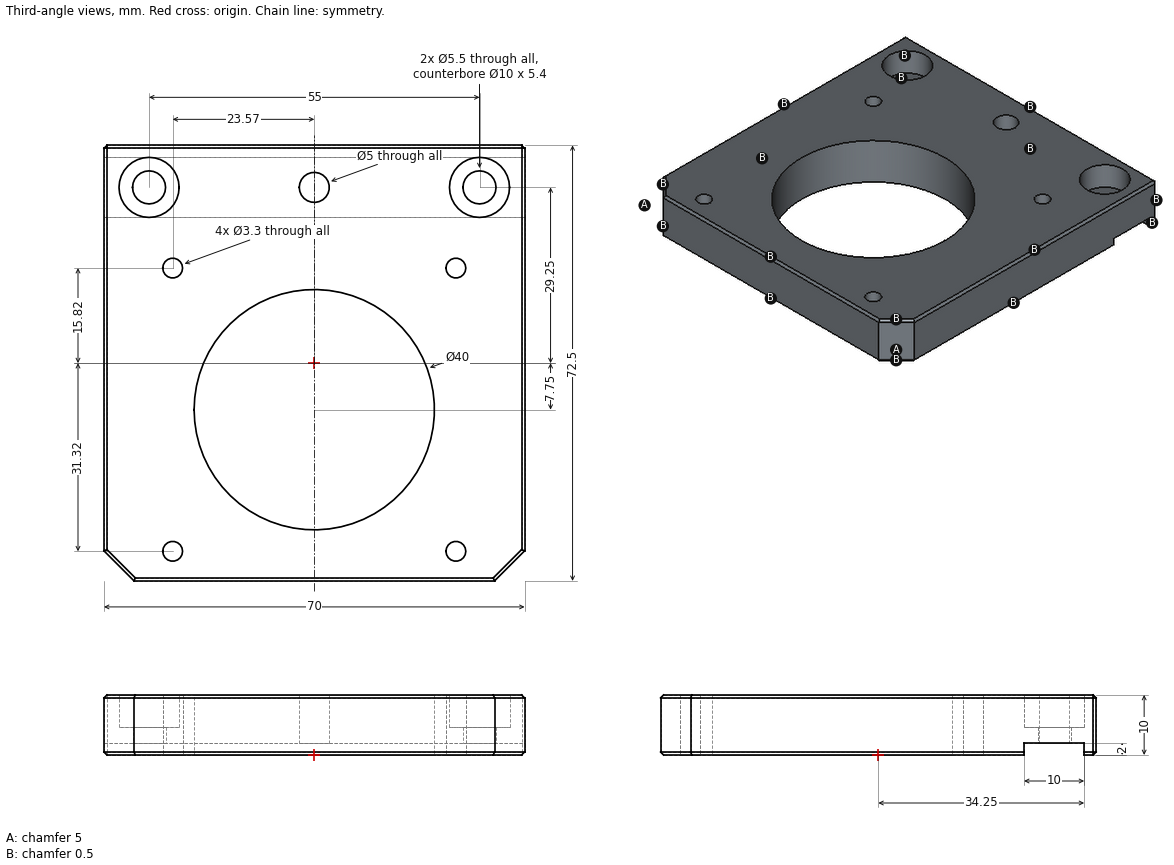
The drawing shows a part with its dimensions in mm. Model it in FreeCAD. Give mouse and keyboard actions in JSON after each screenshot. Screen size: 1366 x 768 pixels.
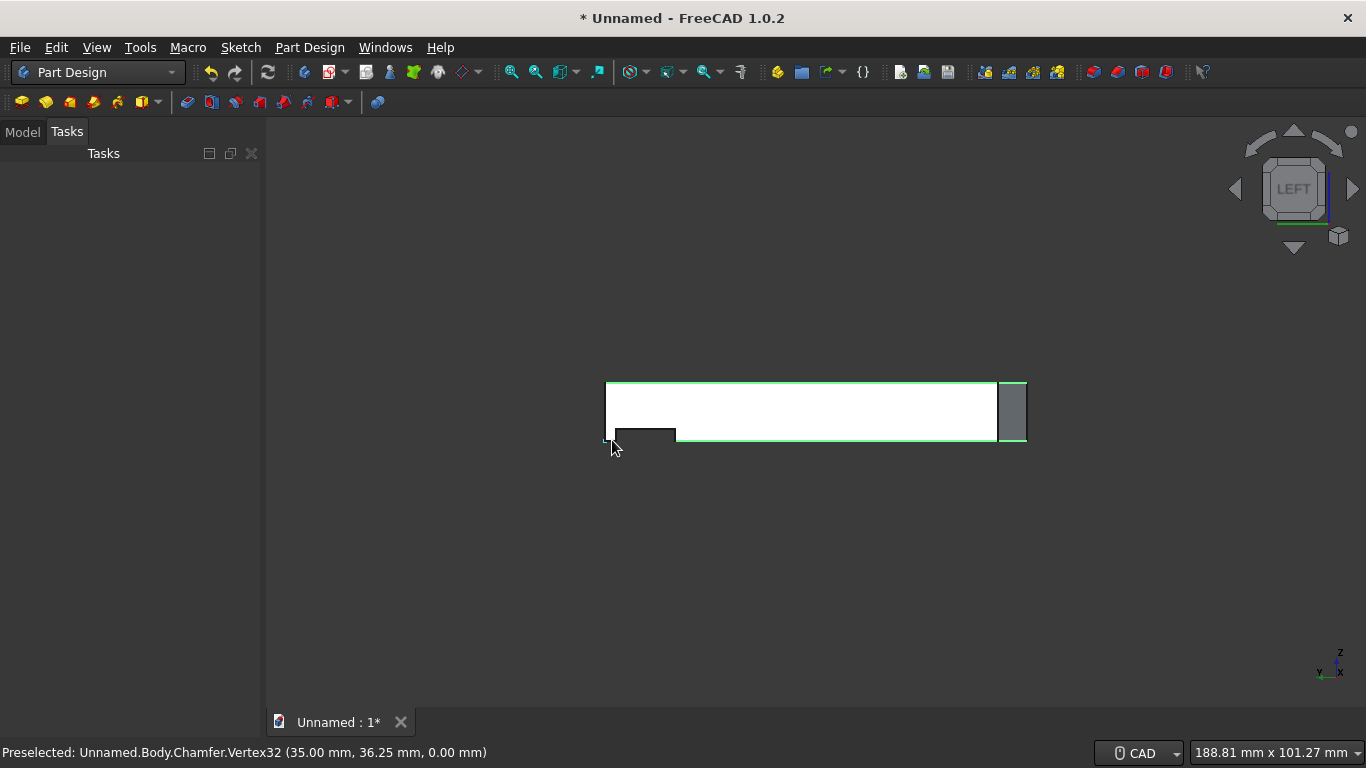
{"action": "left_click", "coordinate": [512, 72]}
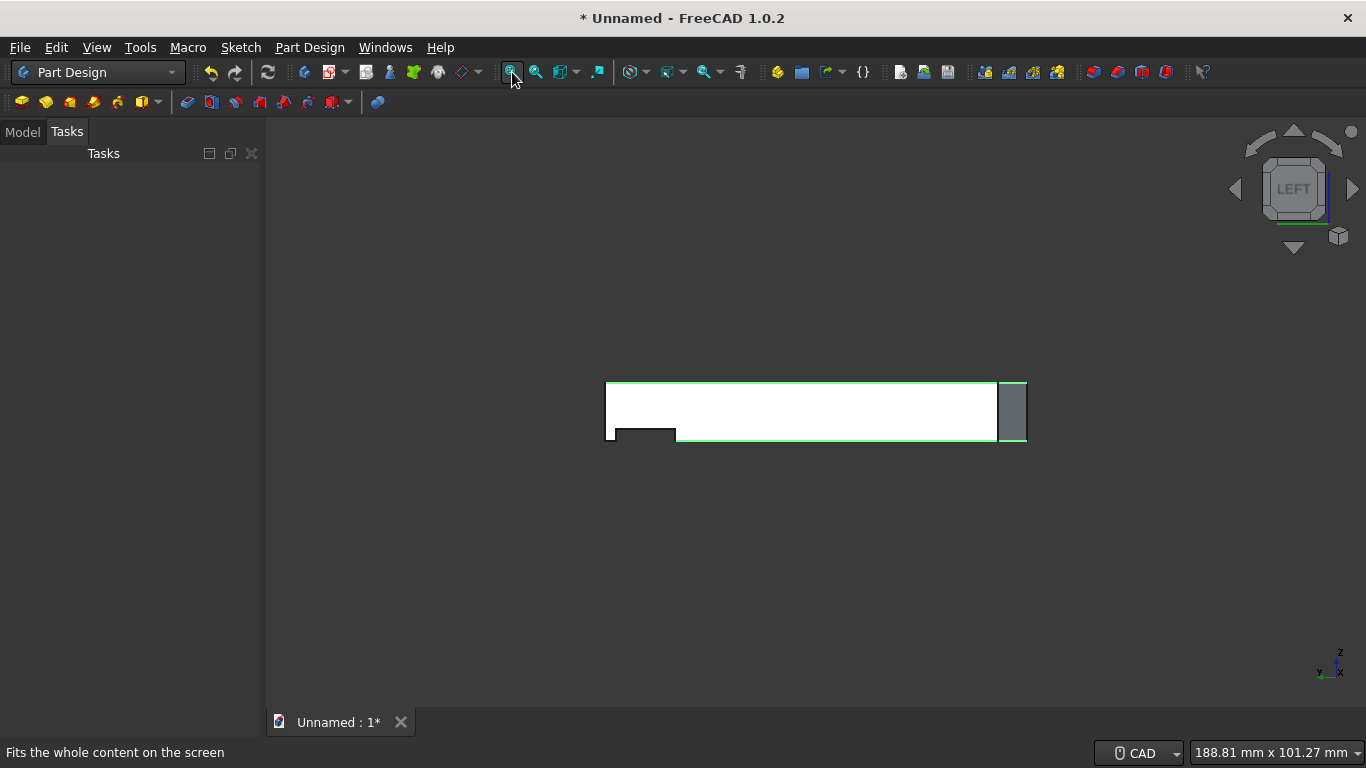
{"action": "scroll", "coordinate": [611, 440], "scroll_direction": "up", "scroll_amount": 7}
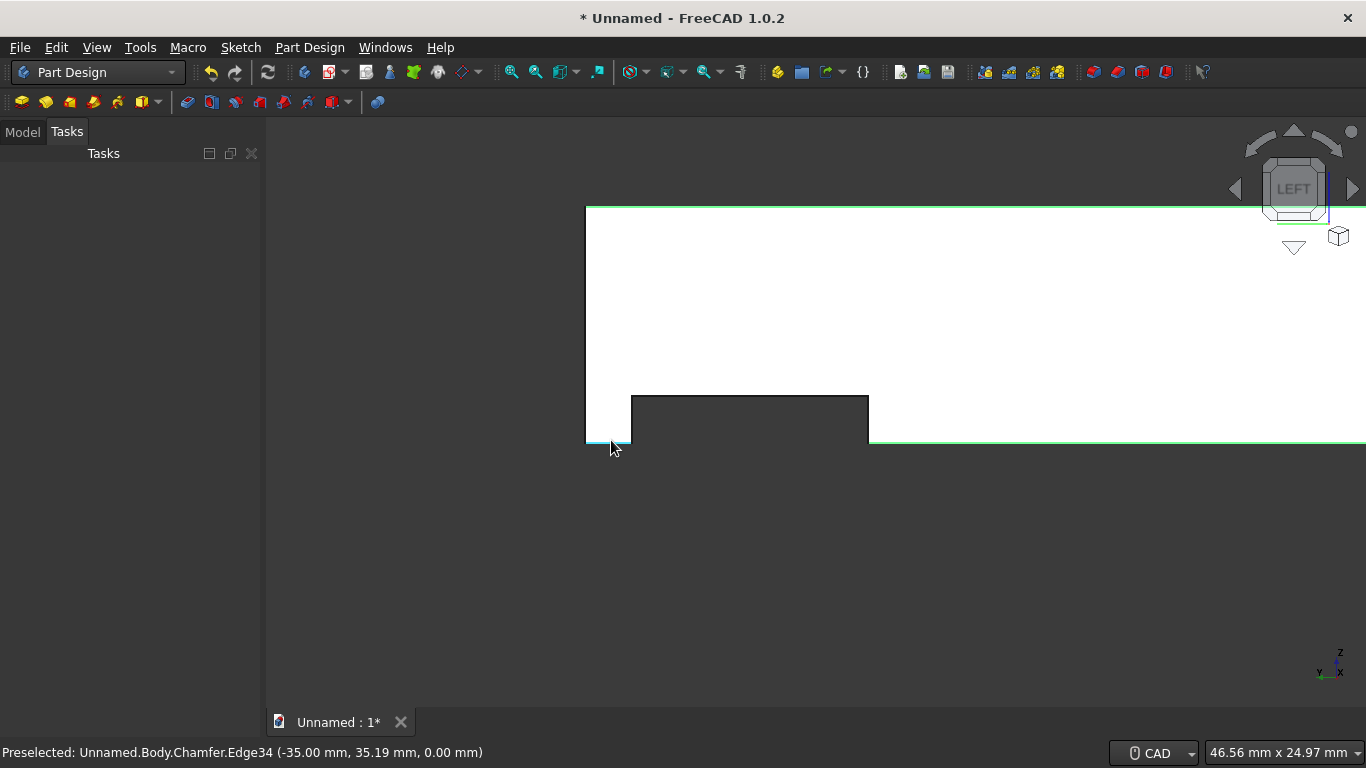
{"action": "left_click", "coordinate": [609, 442], "text": "ctrl"}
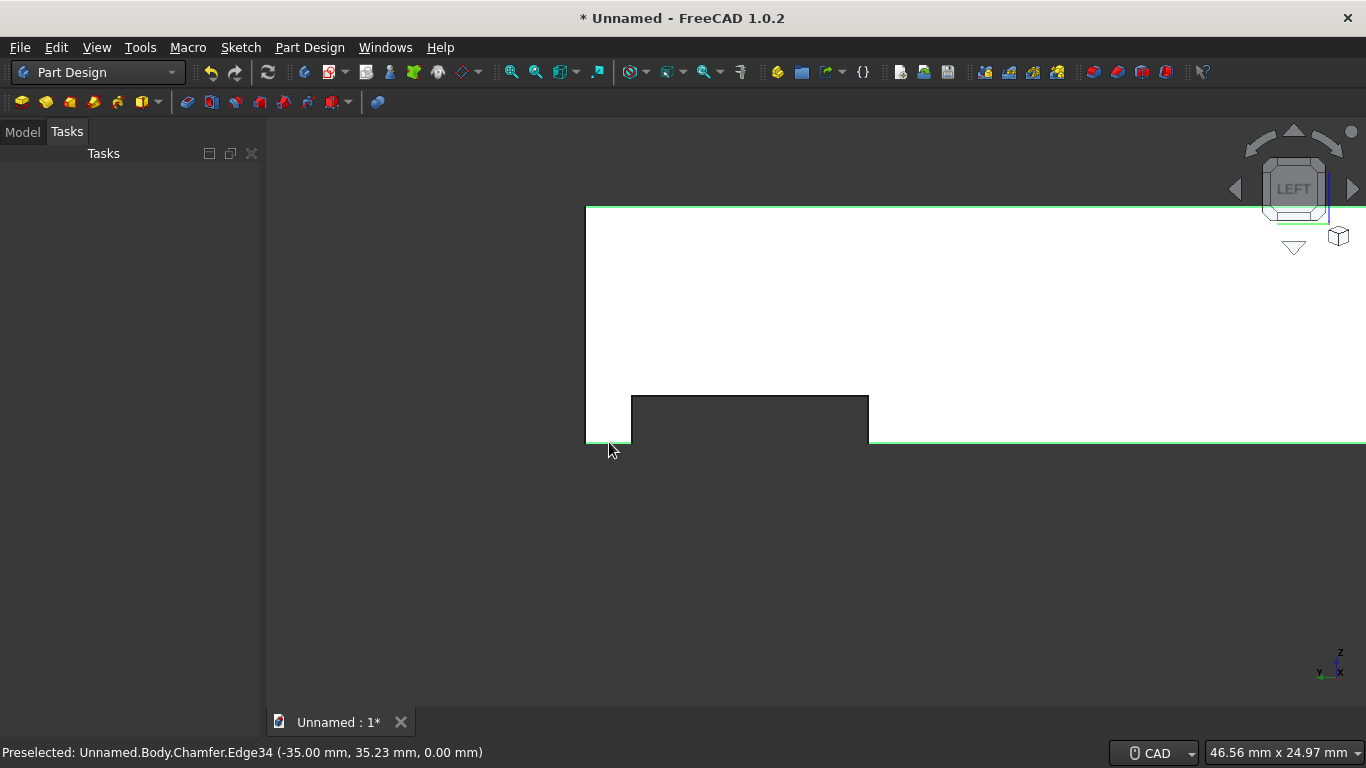
{"action": "left_click", "coordinate": [512, 72]}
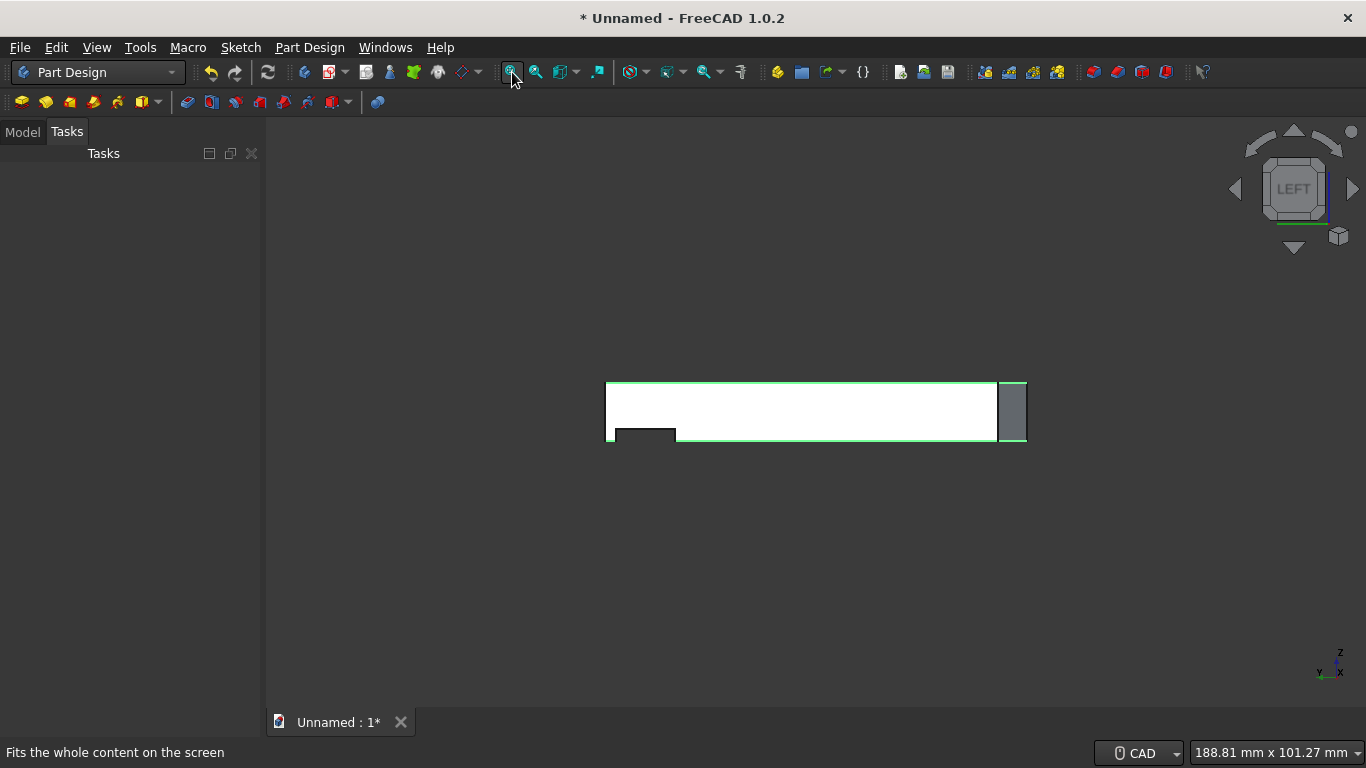
{"action": "key", "text": "v 3"}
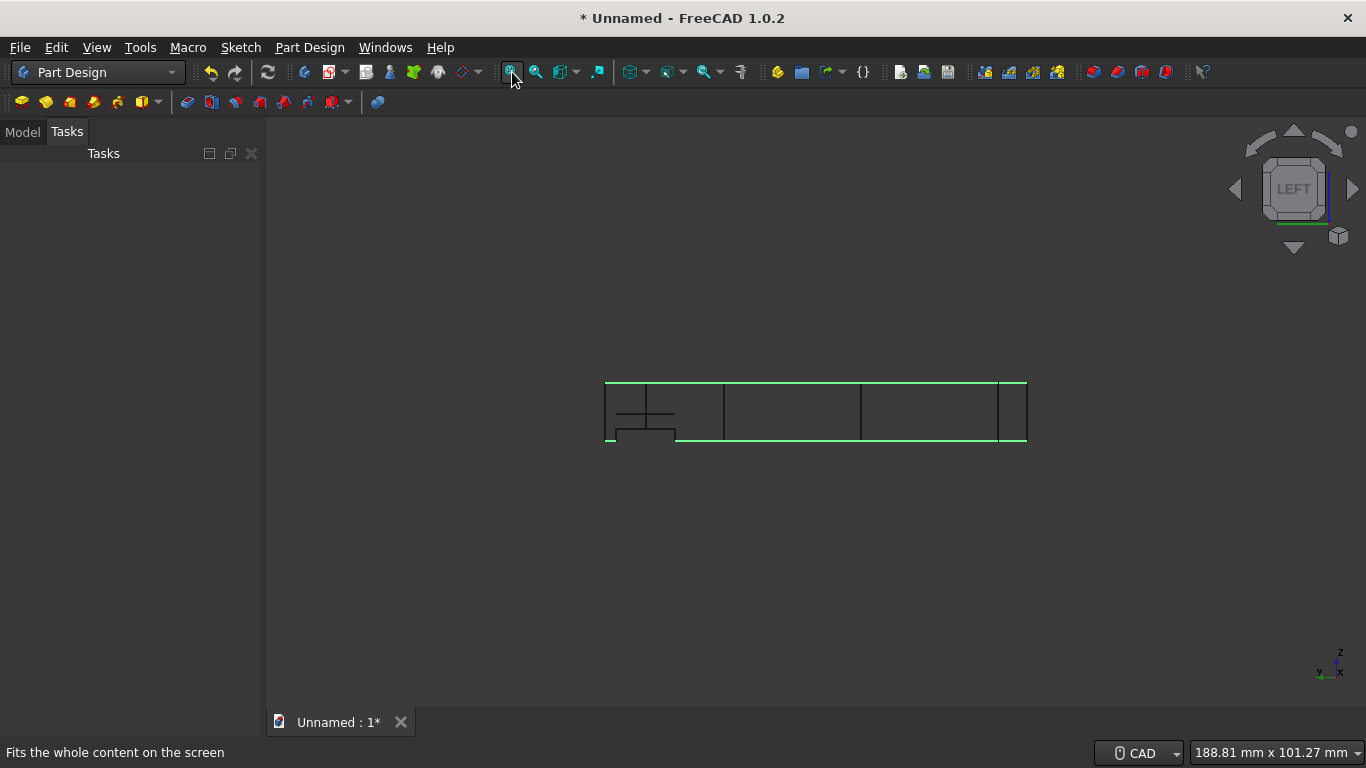
{"action": "key", "text": "0"}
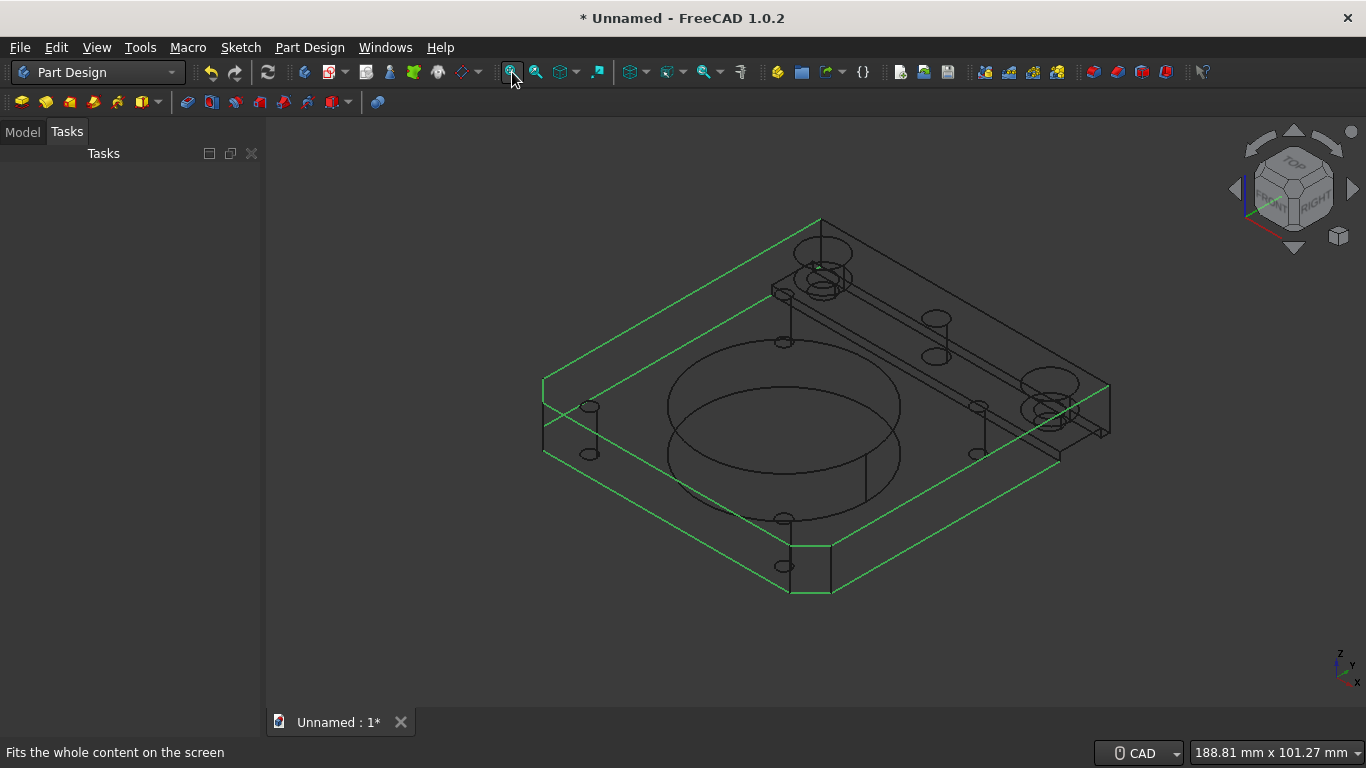
{"action": "scroll", "coordinate": [1105, 434], "scroll_direction": "up", "scroll_amount": 7}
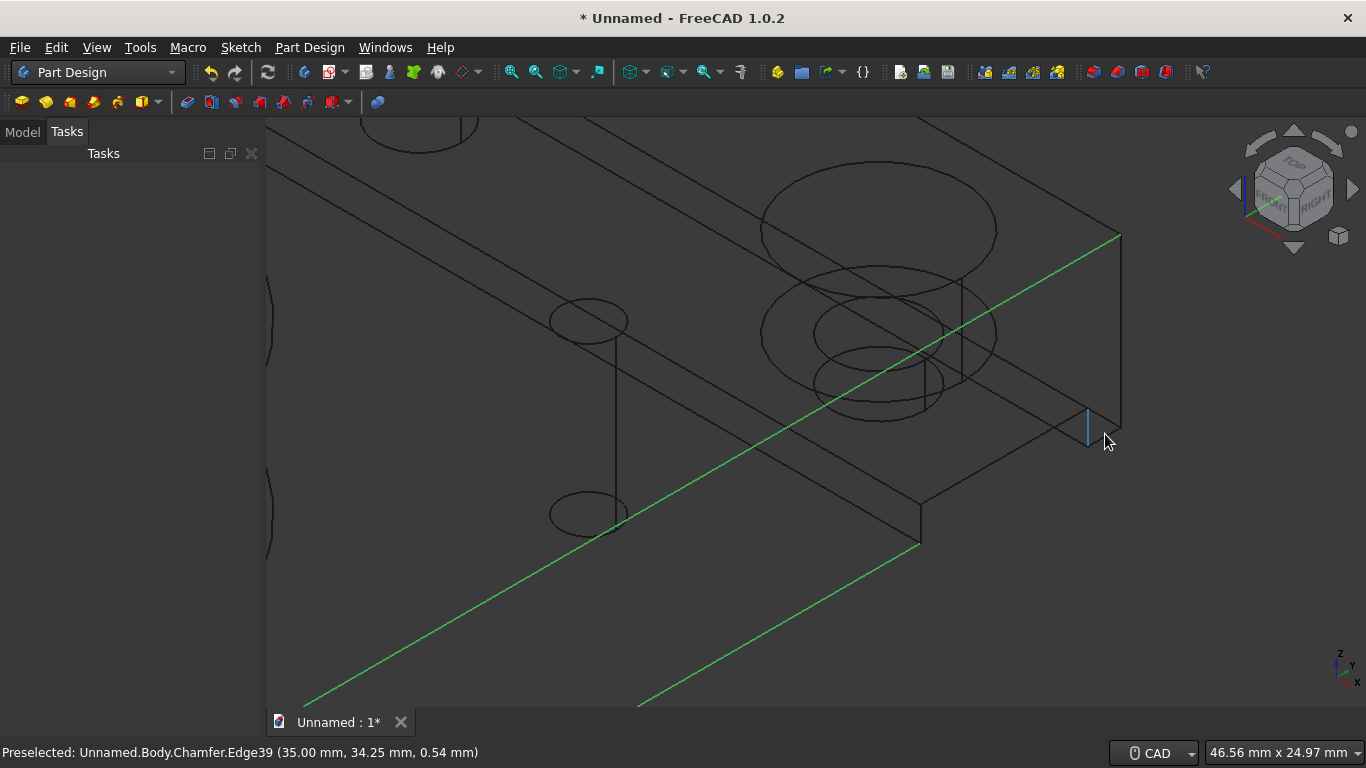
{"action": "left_click", "coordinate": [1104, 436], "text": "ctrl"}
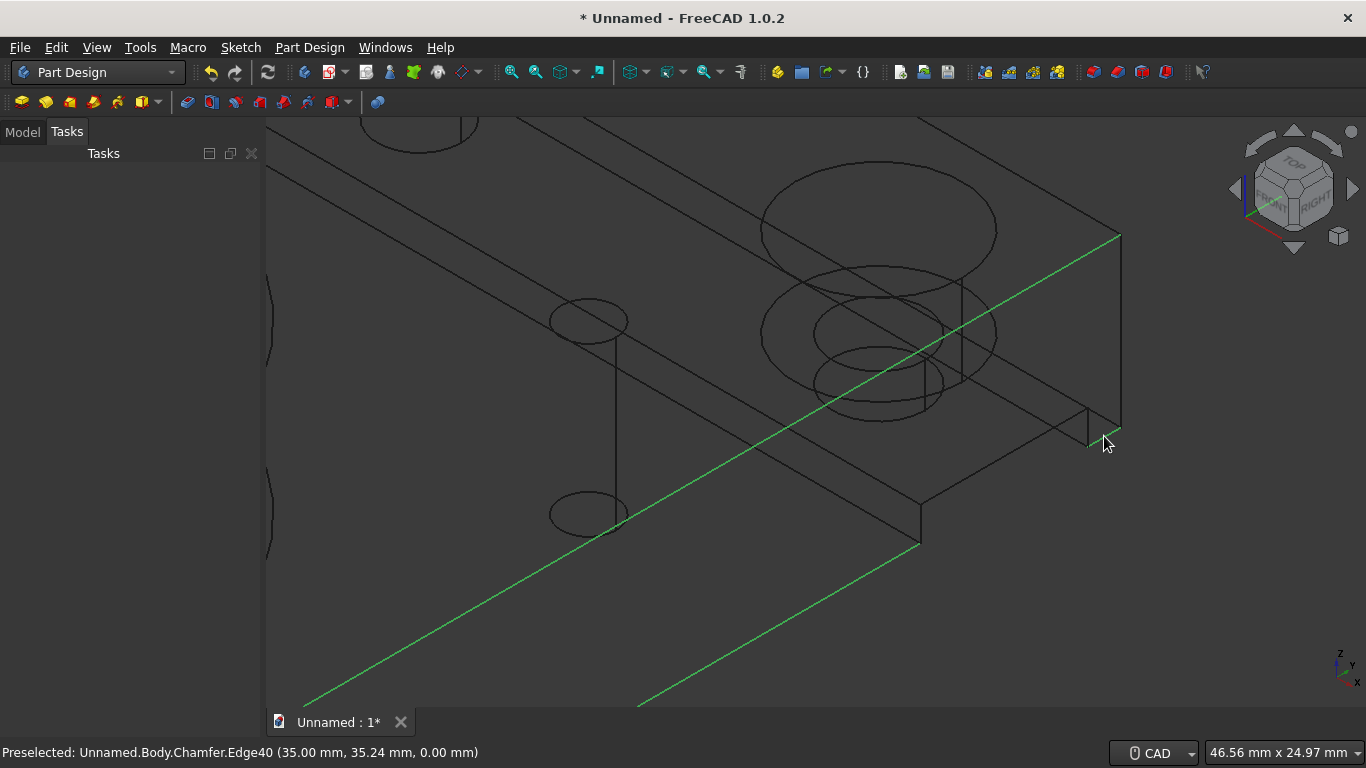
{"action": "key", "text": "v 1"}